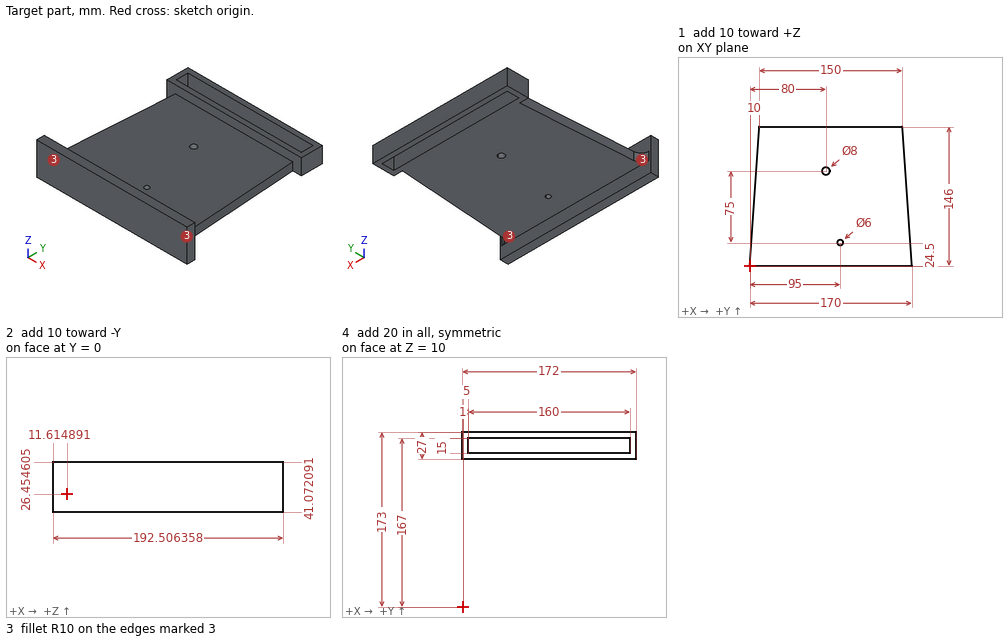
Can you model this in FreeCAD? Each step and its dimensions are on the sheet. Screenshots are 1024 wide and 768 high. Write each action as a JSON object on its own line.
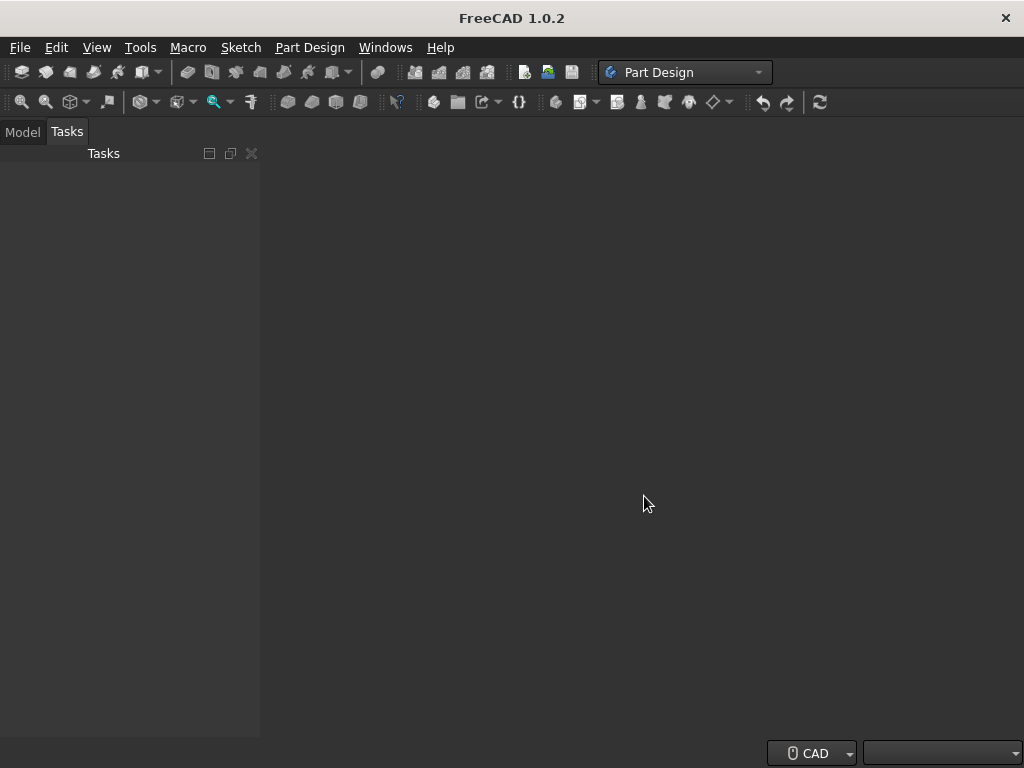
{"action": "key", "text": "ctrl+n"}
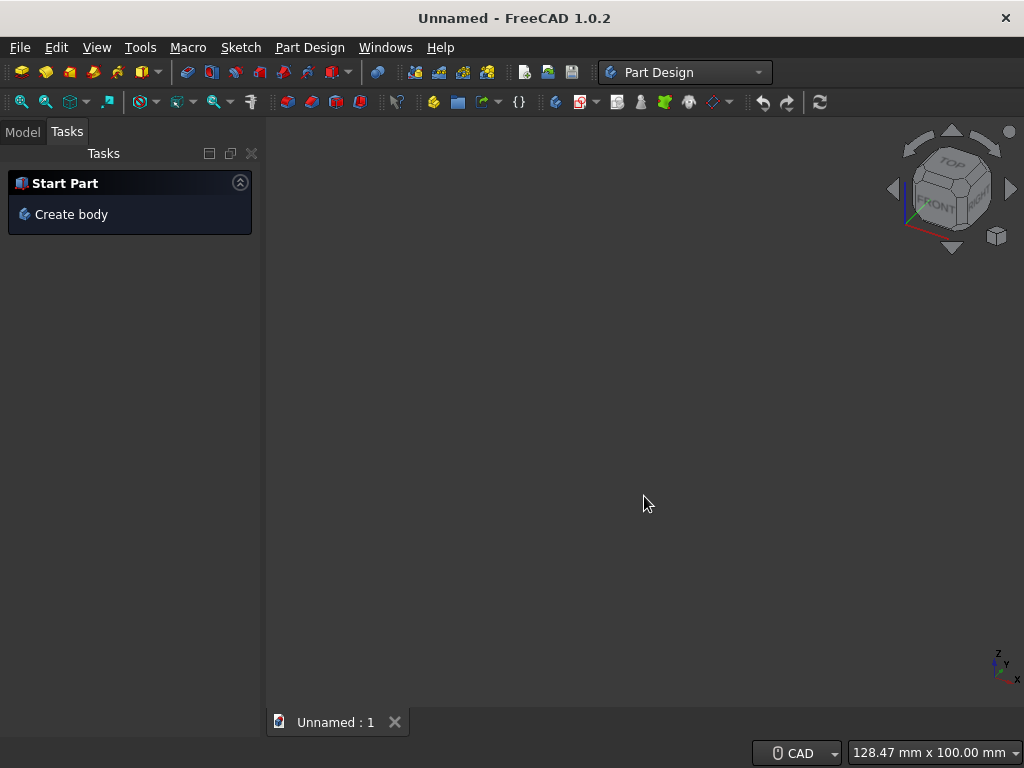
{"action": "left_click", "coordinate": [580, 102]}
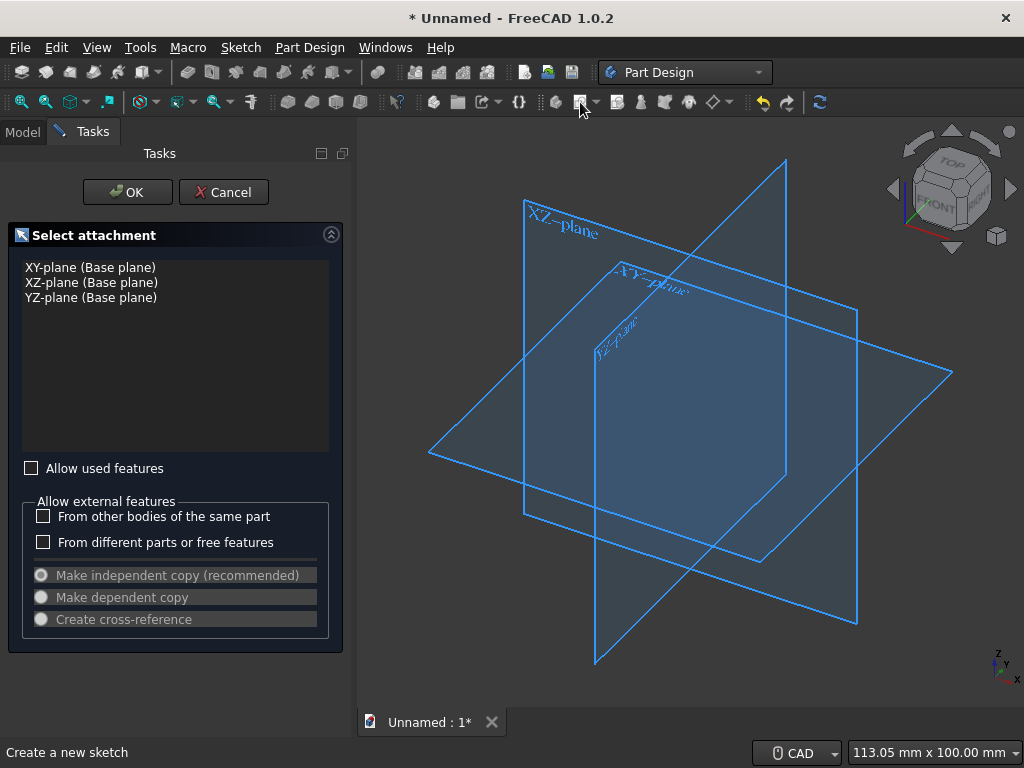
{"action": "left_click", "coordinate": [82, 268]}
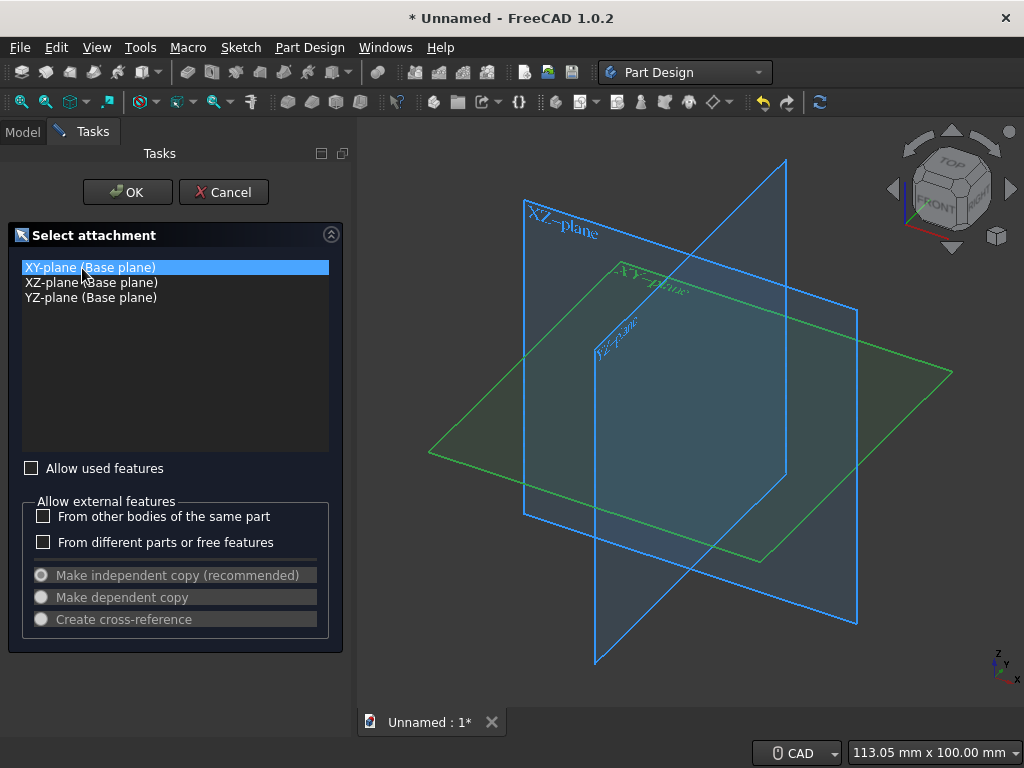
{"action": "left_click", "coordinate": [128, 192]}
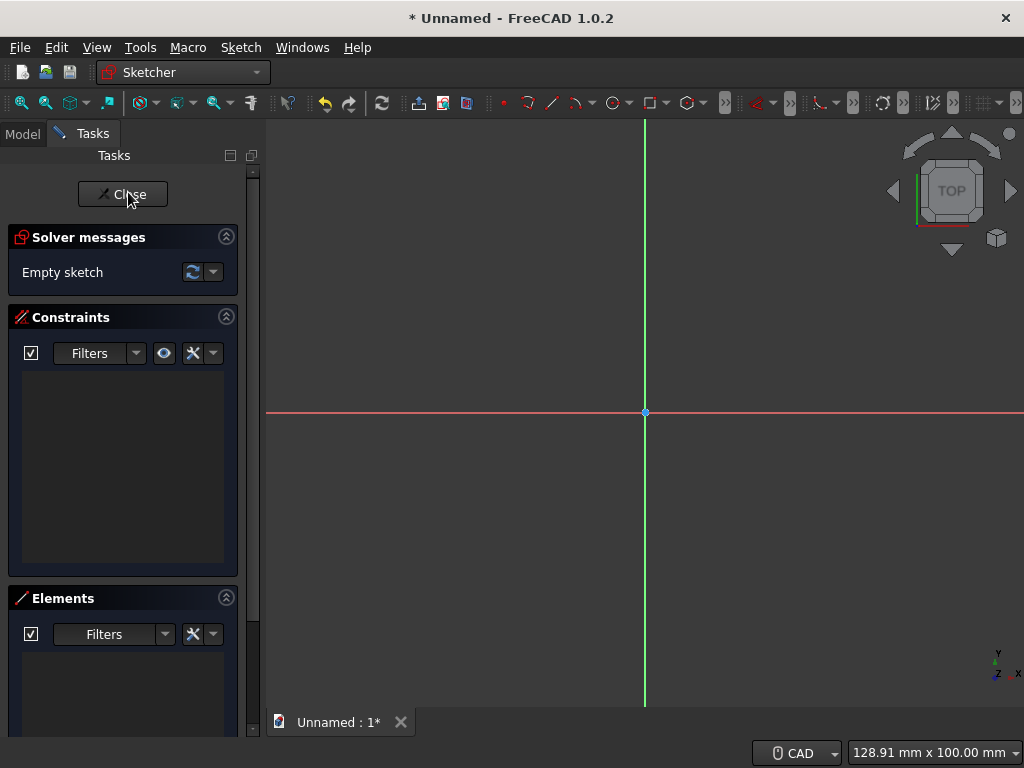
{"action": "scroll", "coordinate": [294, 663], "scroll_direction": "down", "scroll_amount": 5}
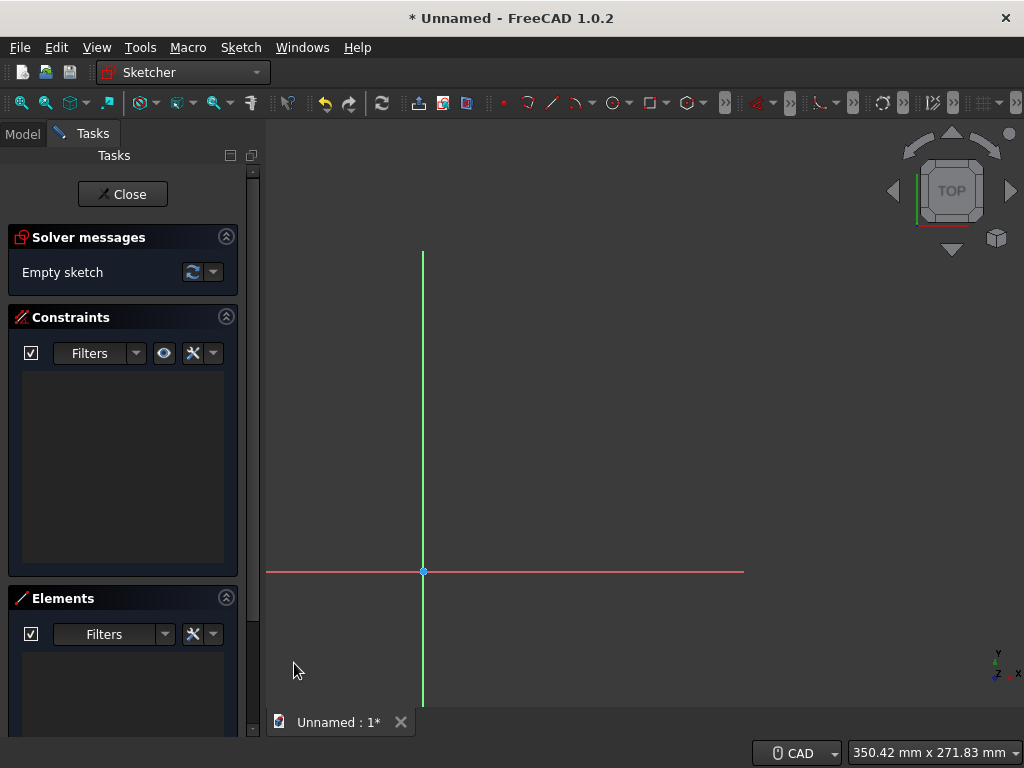
{"action": "left_click", "coordinate": [528, 104]}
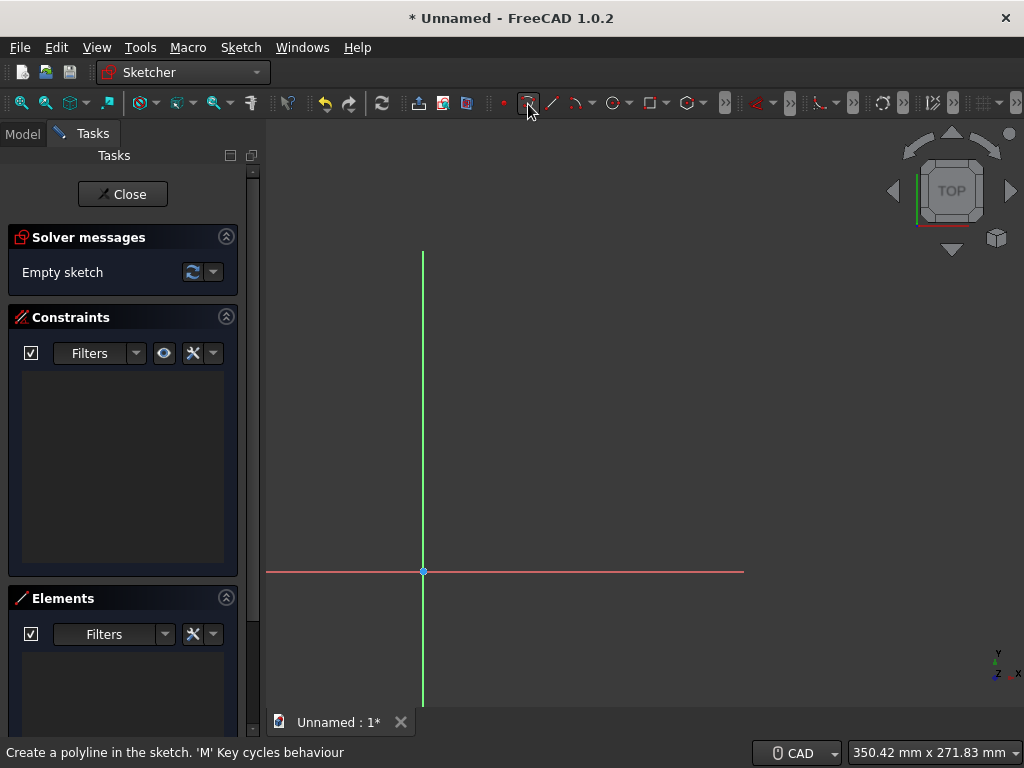
{"action": "left_click", "coordinate": [423, 572]}
{"action": "left_click", "coordinate": [791, 563]}
{"action": "left_click", "coordinate": [769, 256]}
{"action": "left_click", "coordinate": [445, 256]}
{"action": "left_click", "coordinate": [423, 572]}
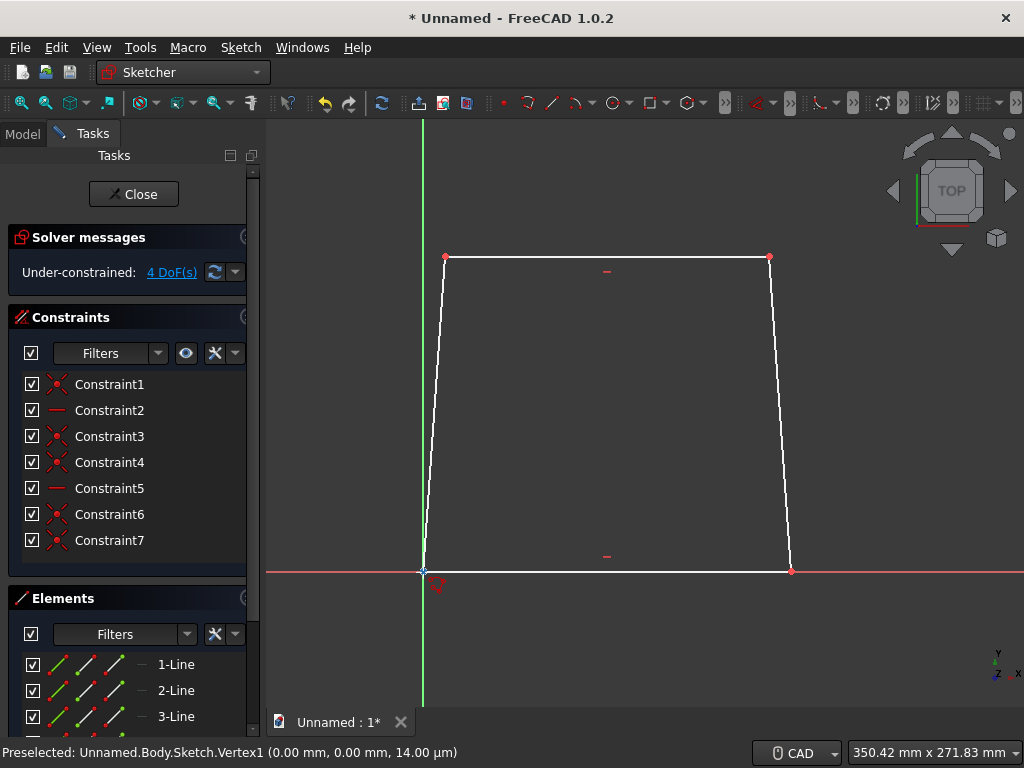
{"action": "key", "text": "g c"}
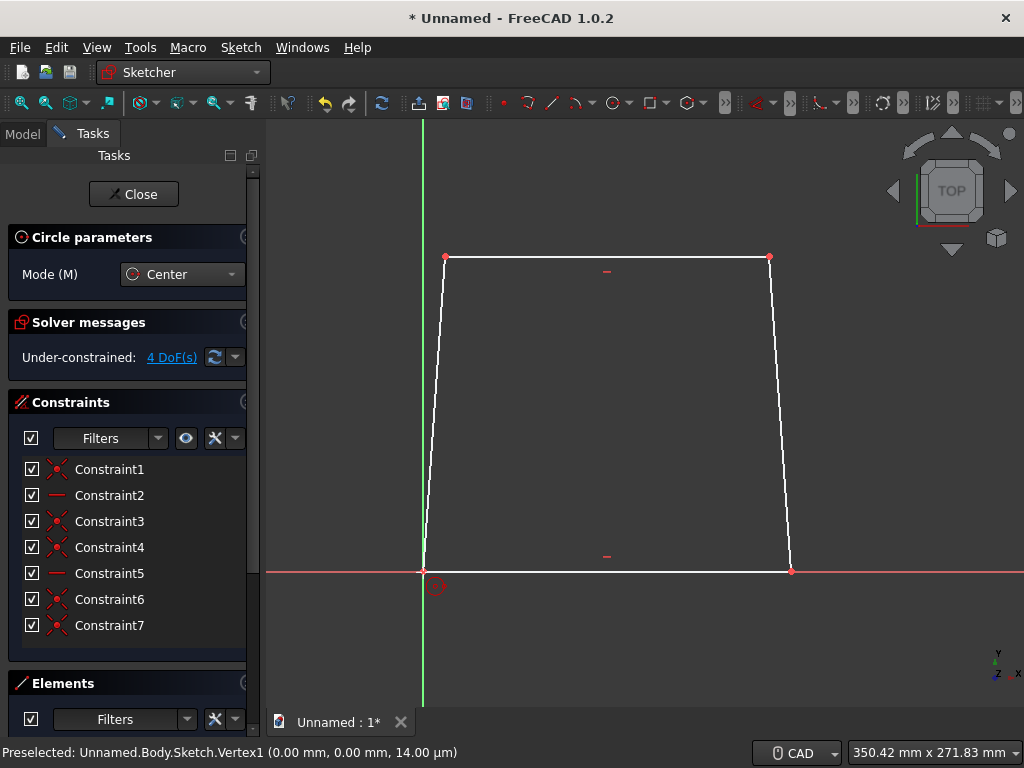
{"action": "scroll", "coordinate": [629, 519], "scroll_direction": "up", "scroll_amount": 7}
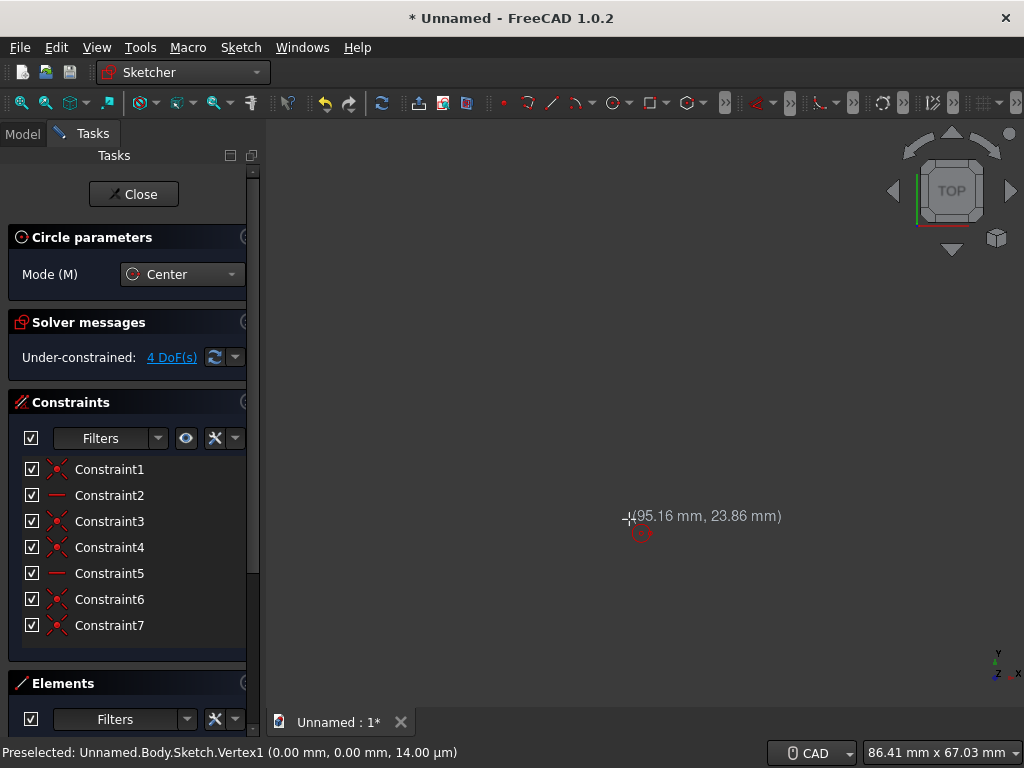
{"action": "scroll", "coordinate": [589, 519], "scroll_direction": "down", "scroll_amount": 7}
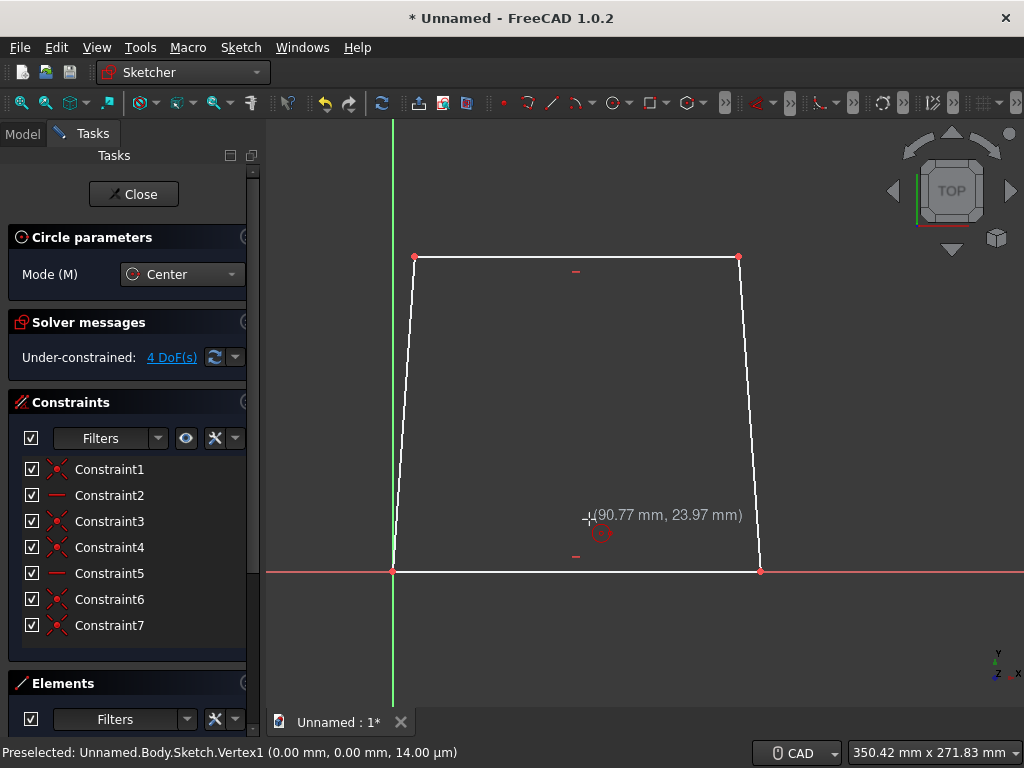
{"action": "left_click", "coordinate": [598, 519]}
{"action": "mouse_move", "coordinate": [603, 514]}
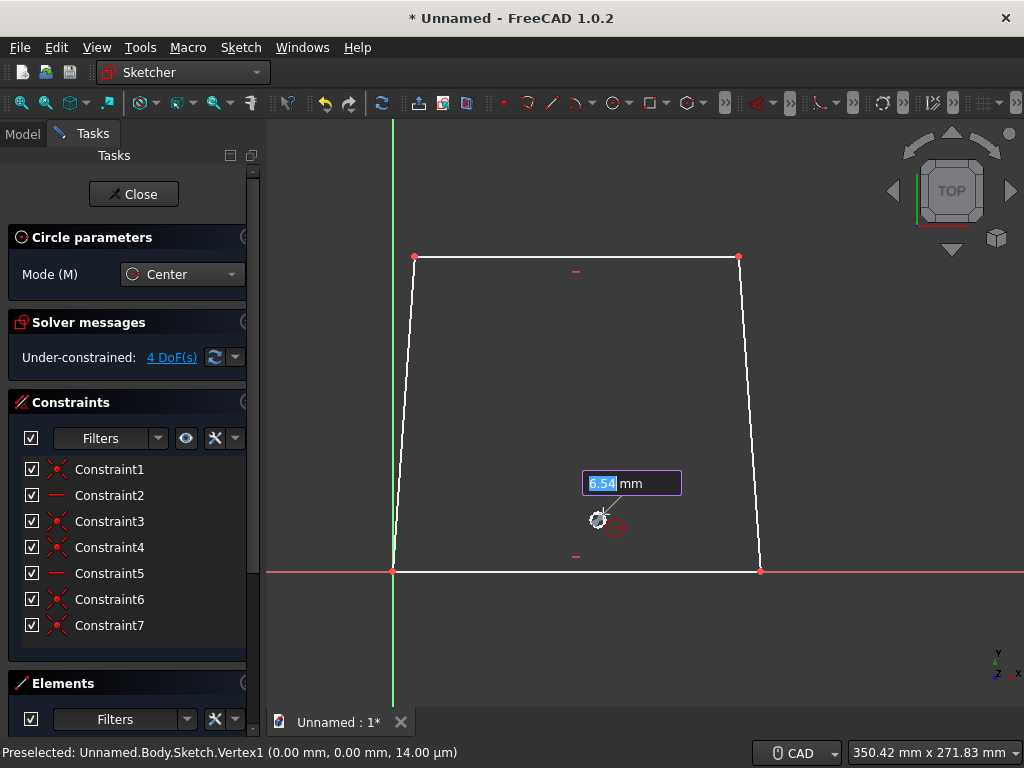
{"action": "type", "text": "6"}
{"action": "key", "text": "Return"}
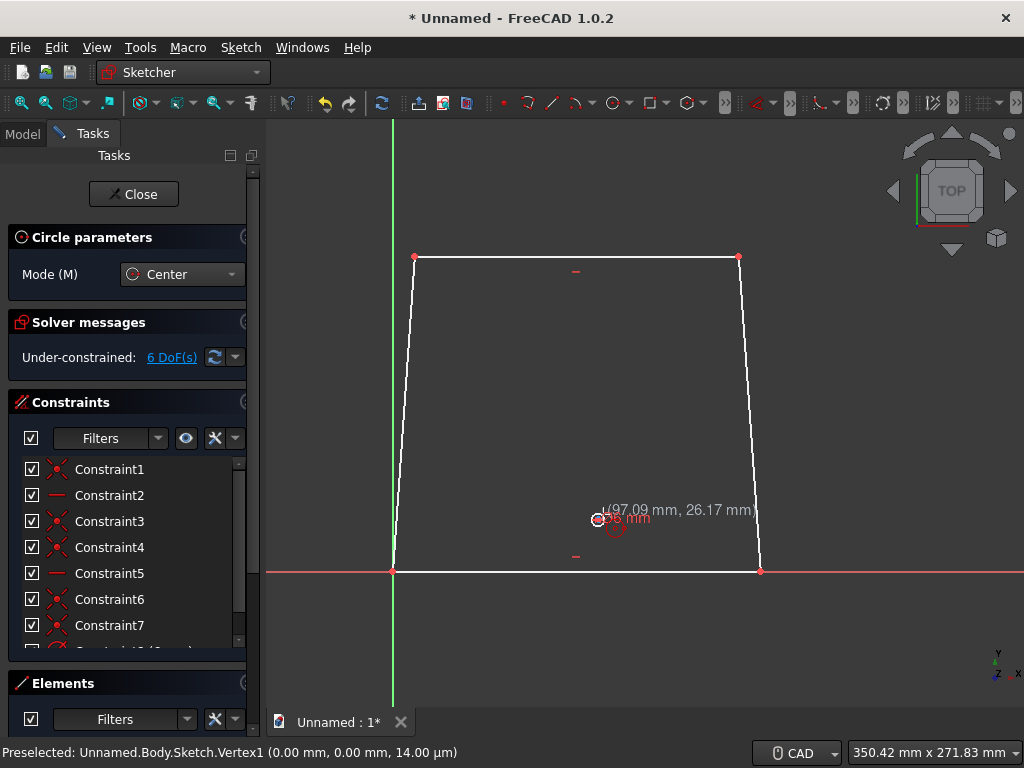
{"action": "scroll", "coordinate": [566, 356], "scroll_direction": "up", "scroll_amount": 5}